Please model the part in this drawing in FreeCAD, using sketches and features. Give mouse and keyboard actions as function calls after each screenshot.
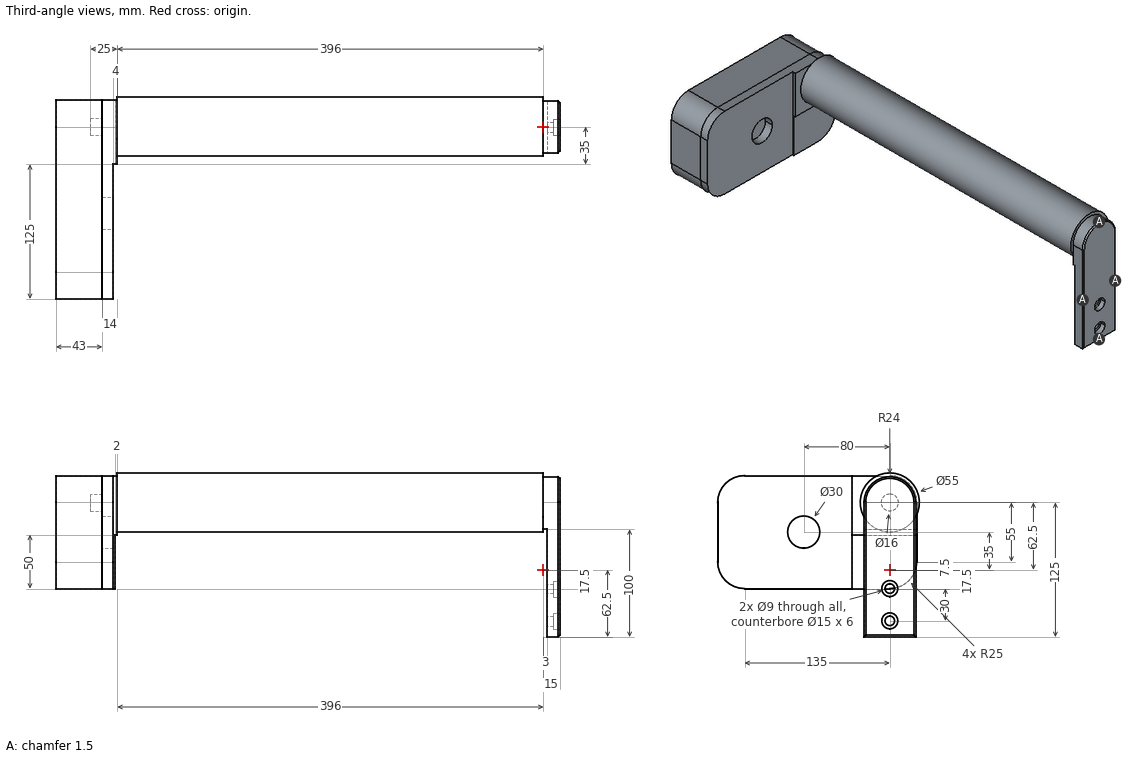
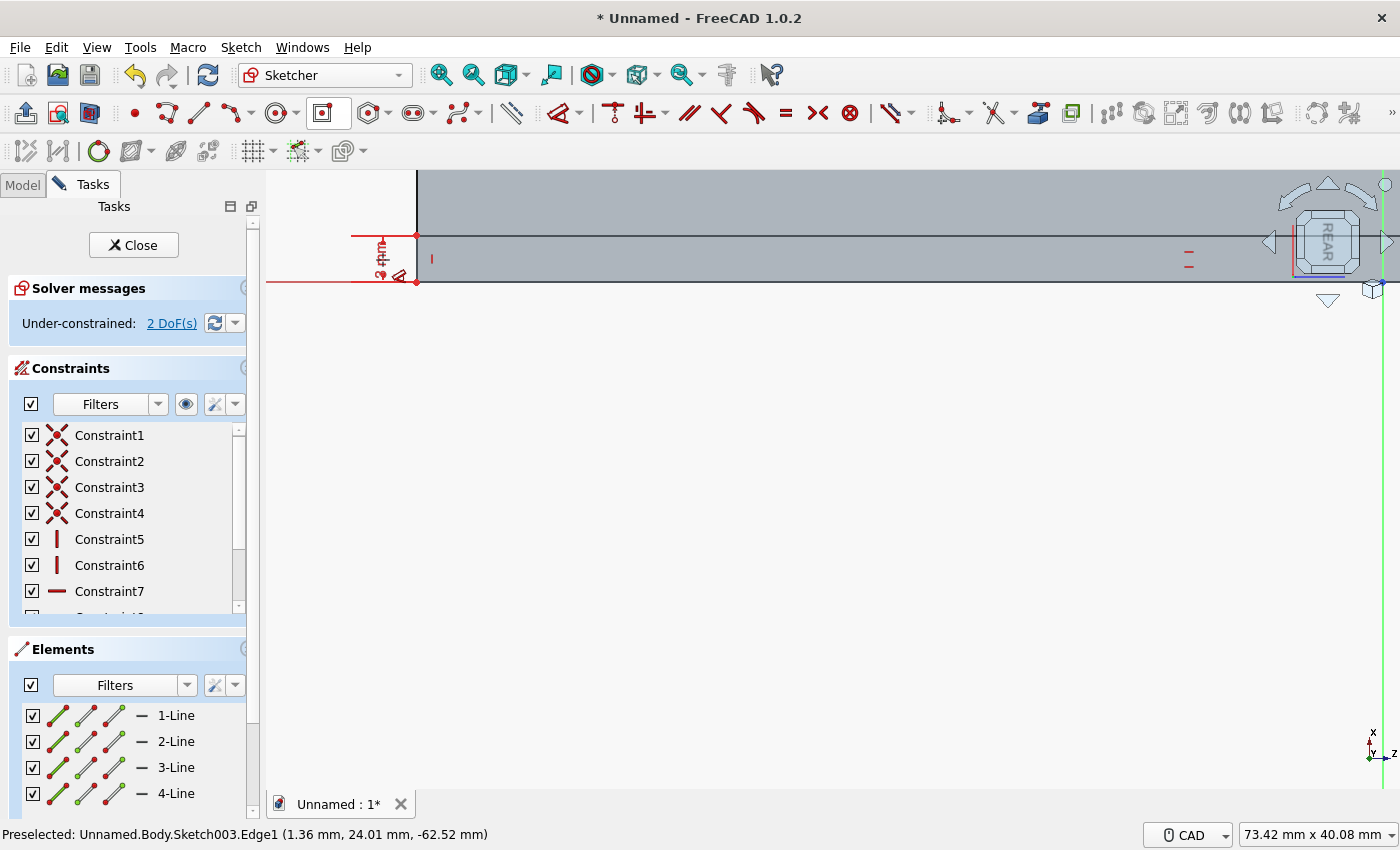
click(880, 282)
click(826, 316)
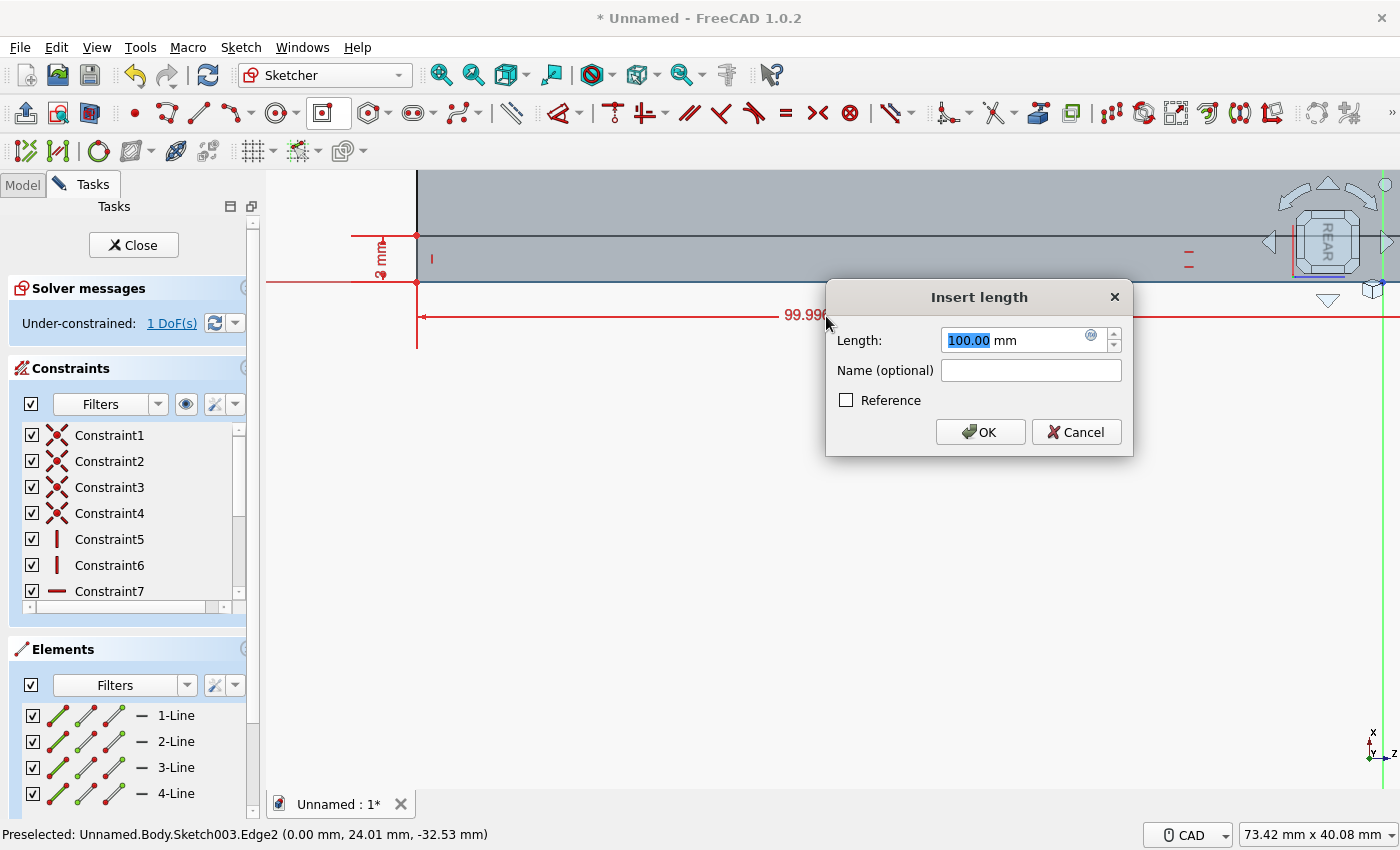
text(100)
key(Return)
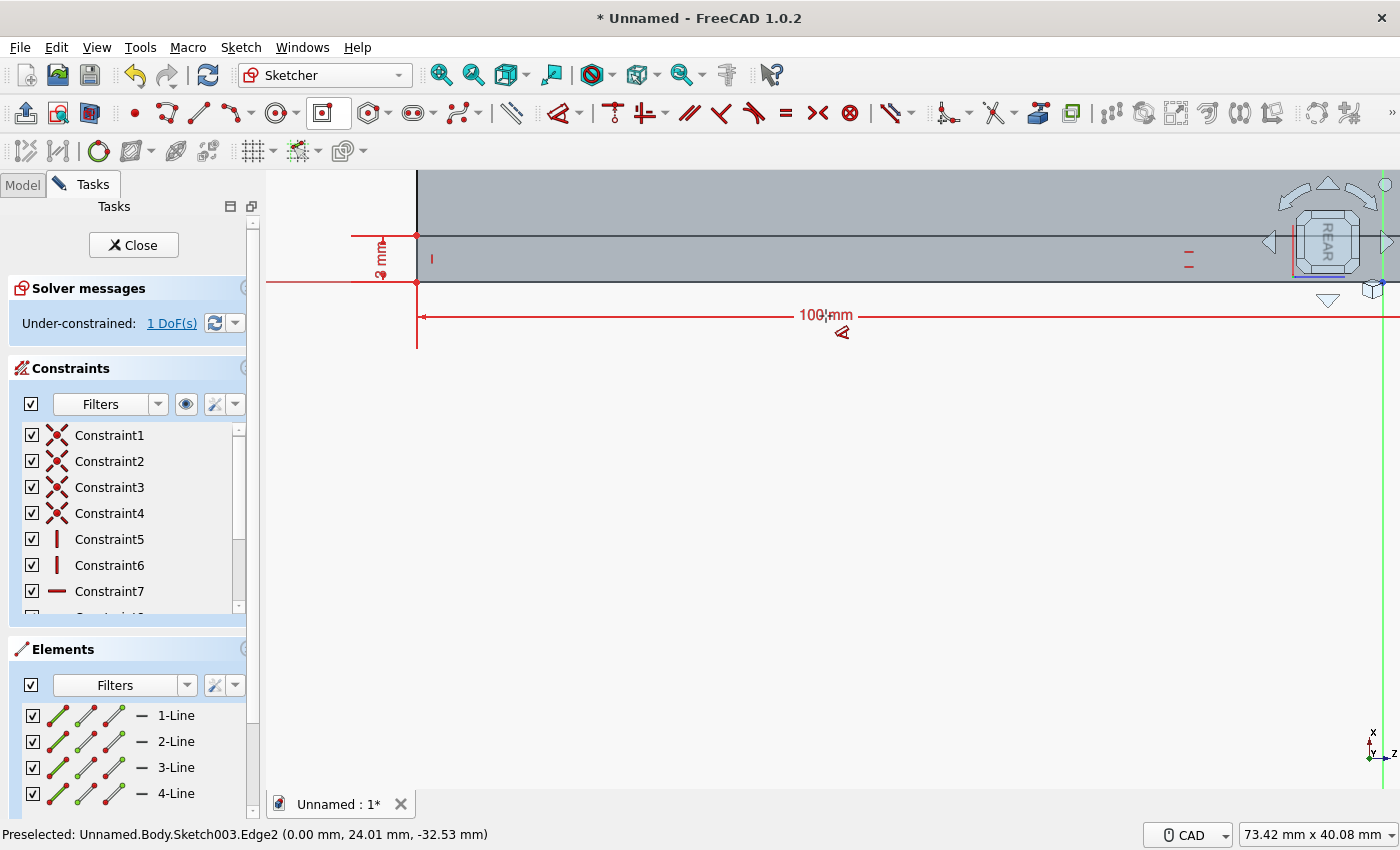
click(417, 236)
click(638, 316)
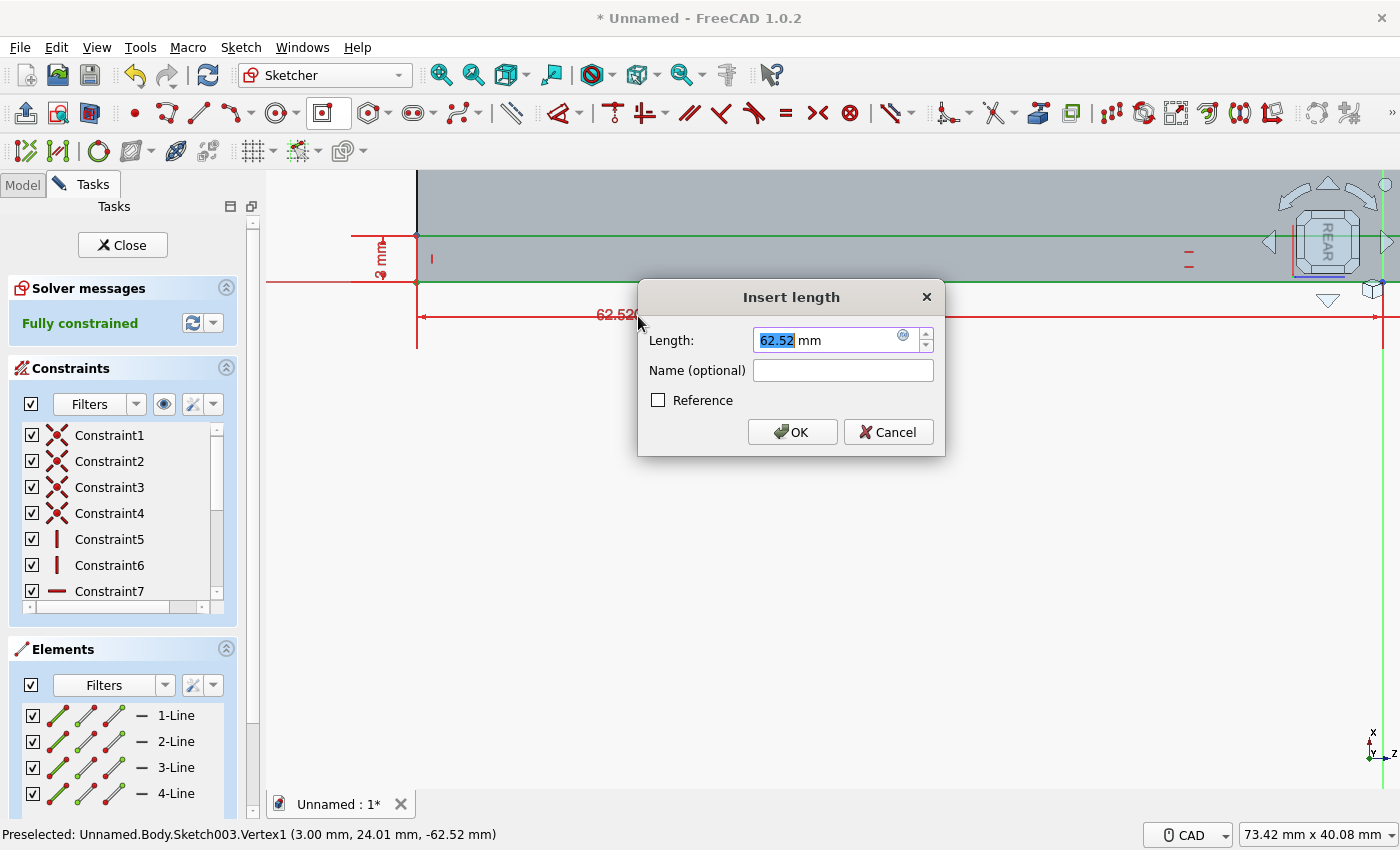
text(62.5)
key(Return)
key(Escape)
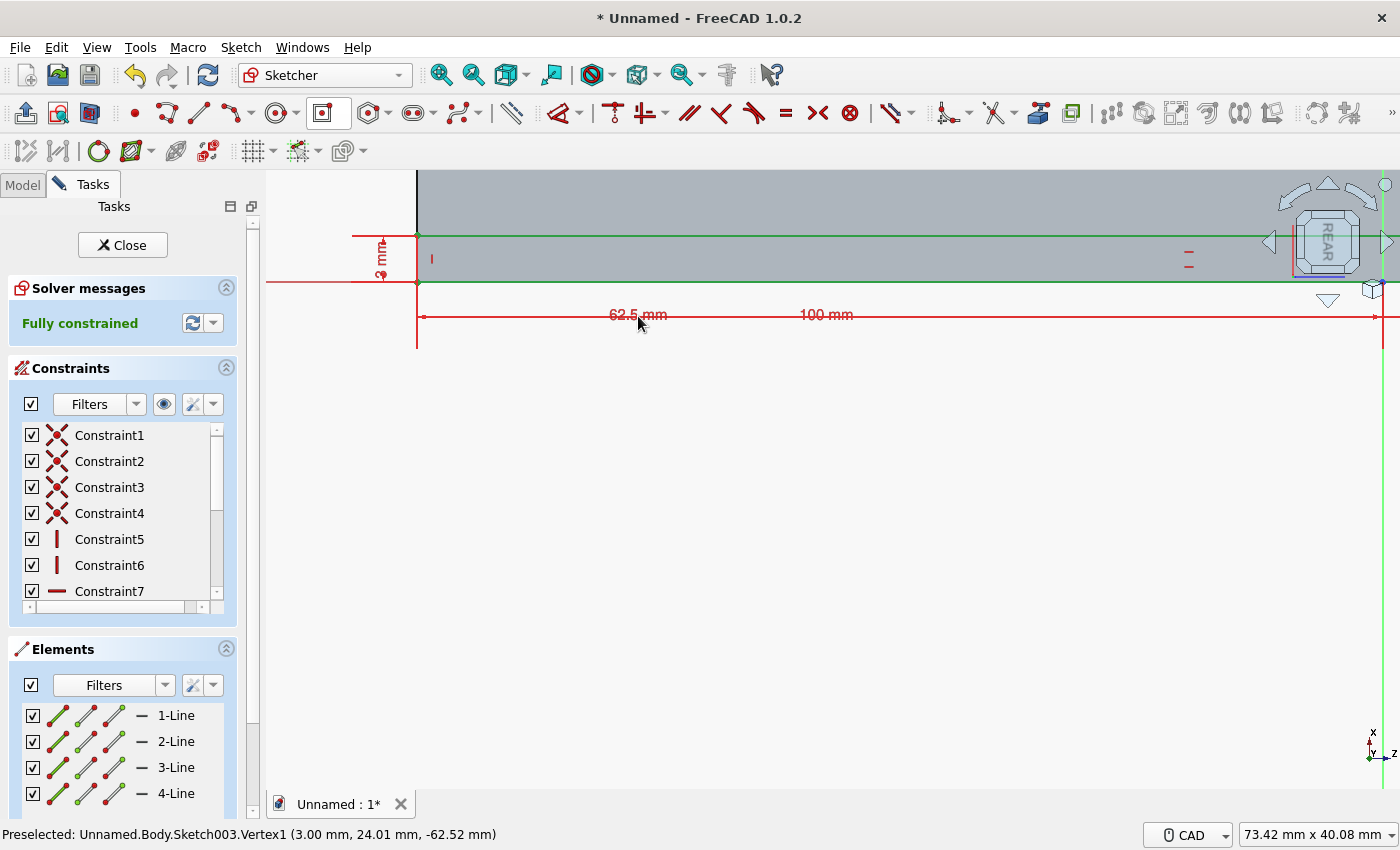
click(123, 245)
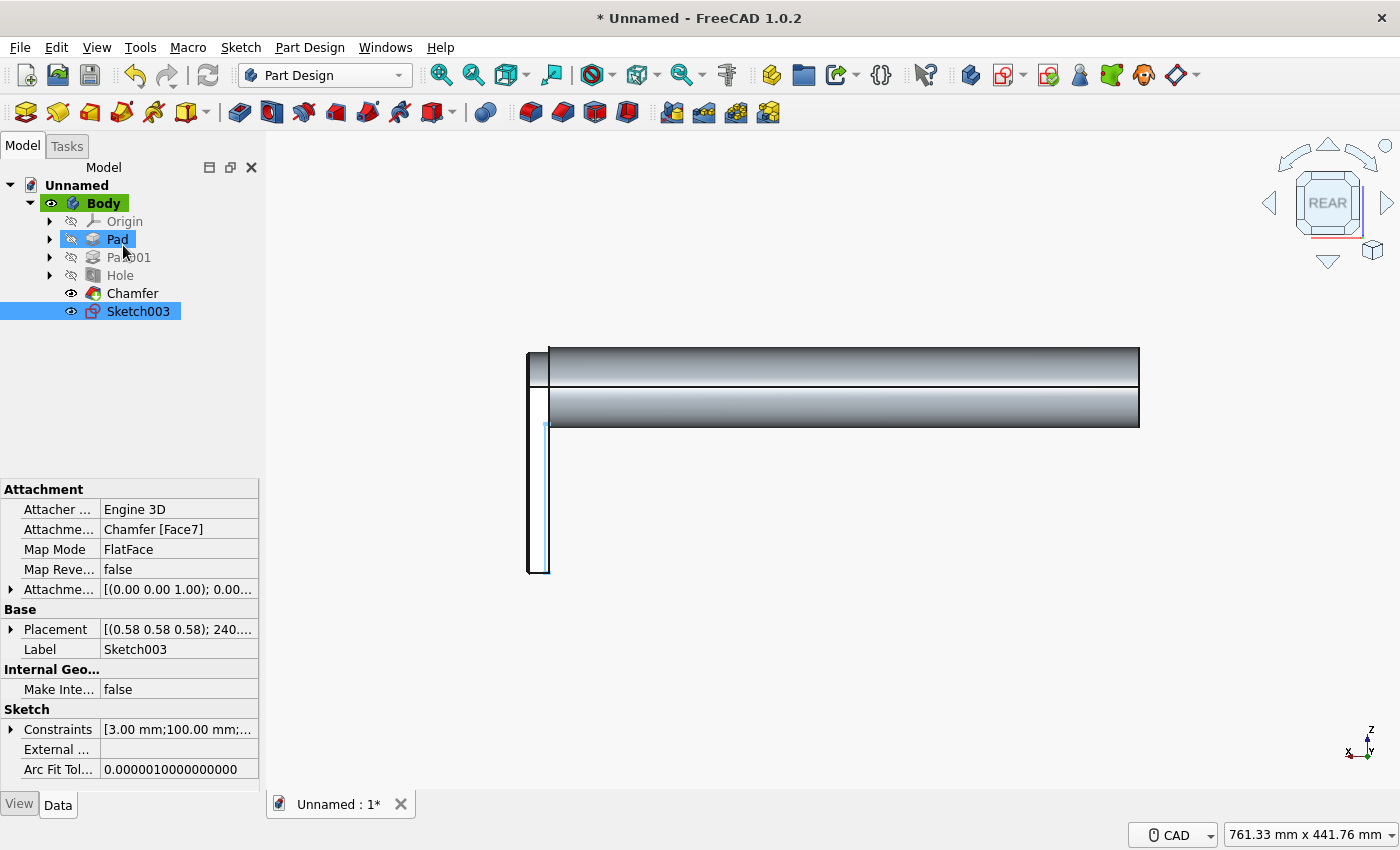
click(240, 112)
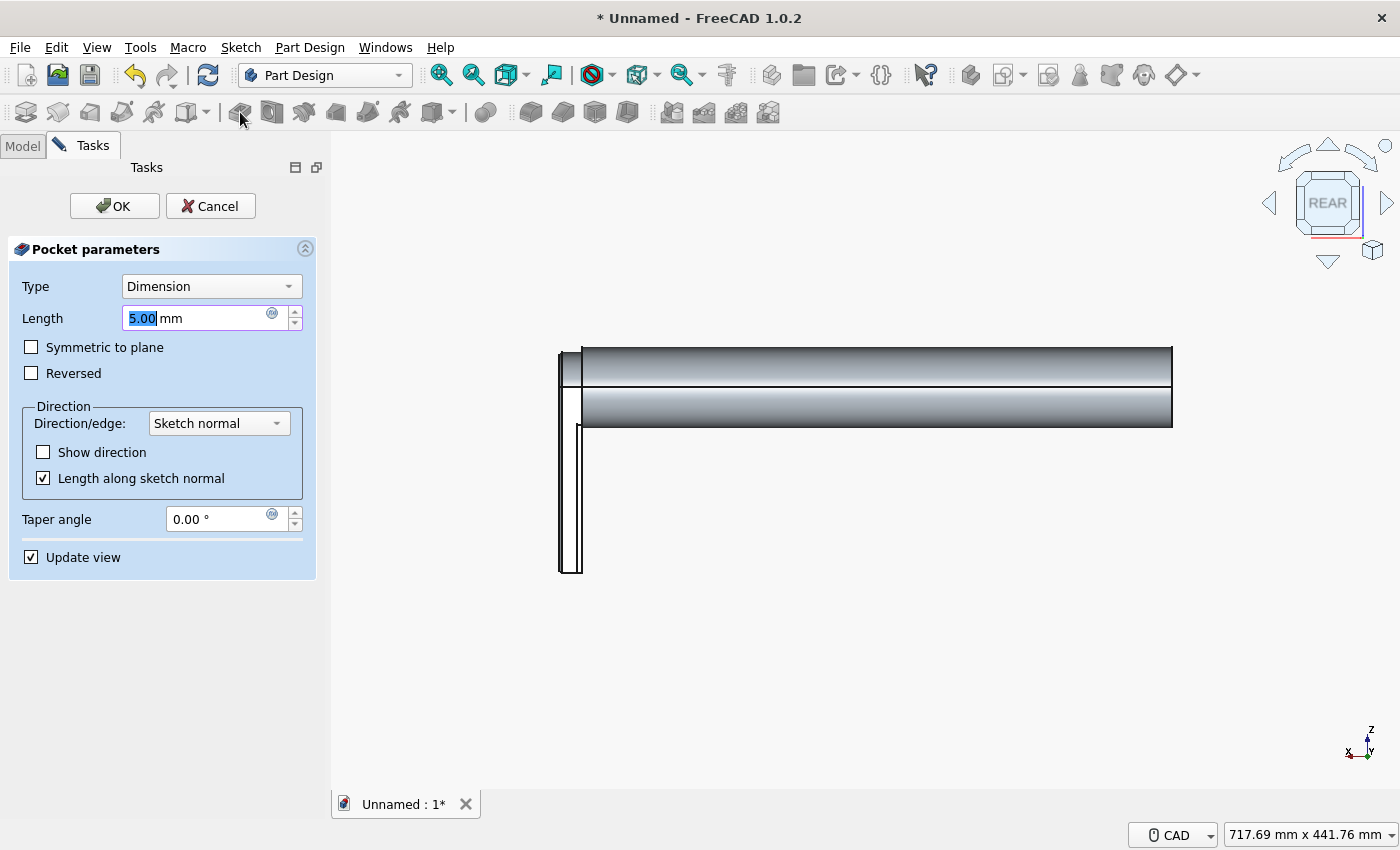
click(212, 286)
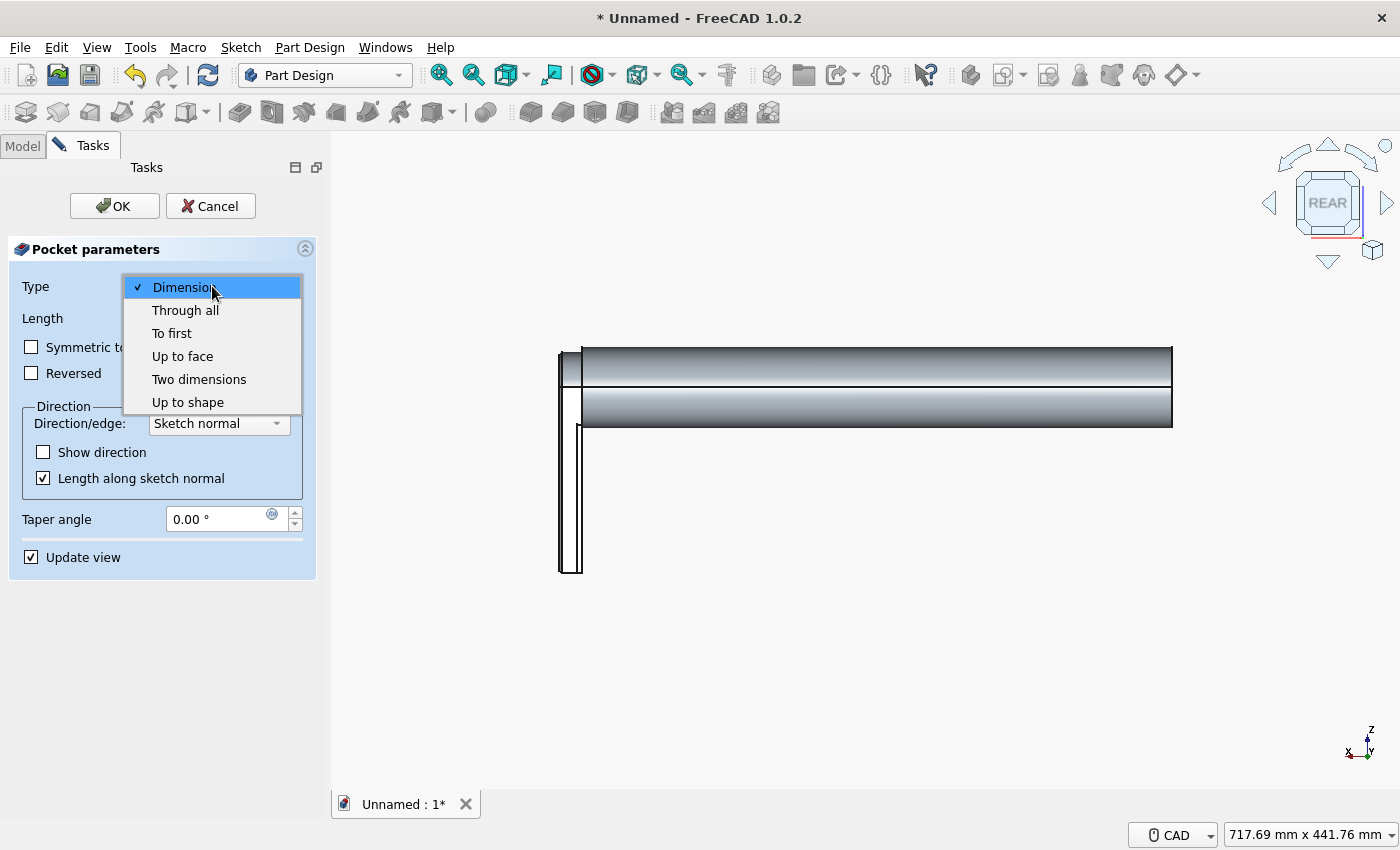
click(212, 310)